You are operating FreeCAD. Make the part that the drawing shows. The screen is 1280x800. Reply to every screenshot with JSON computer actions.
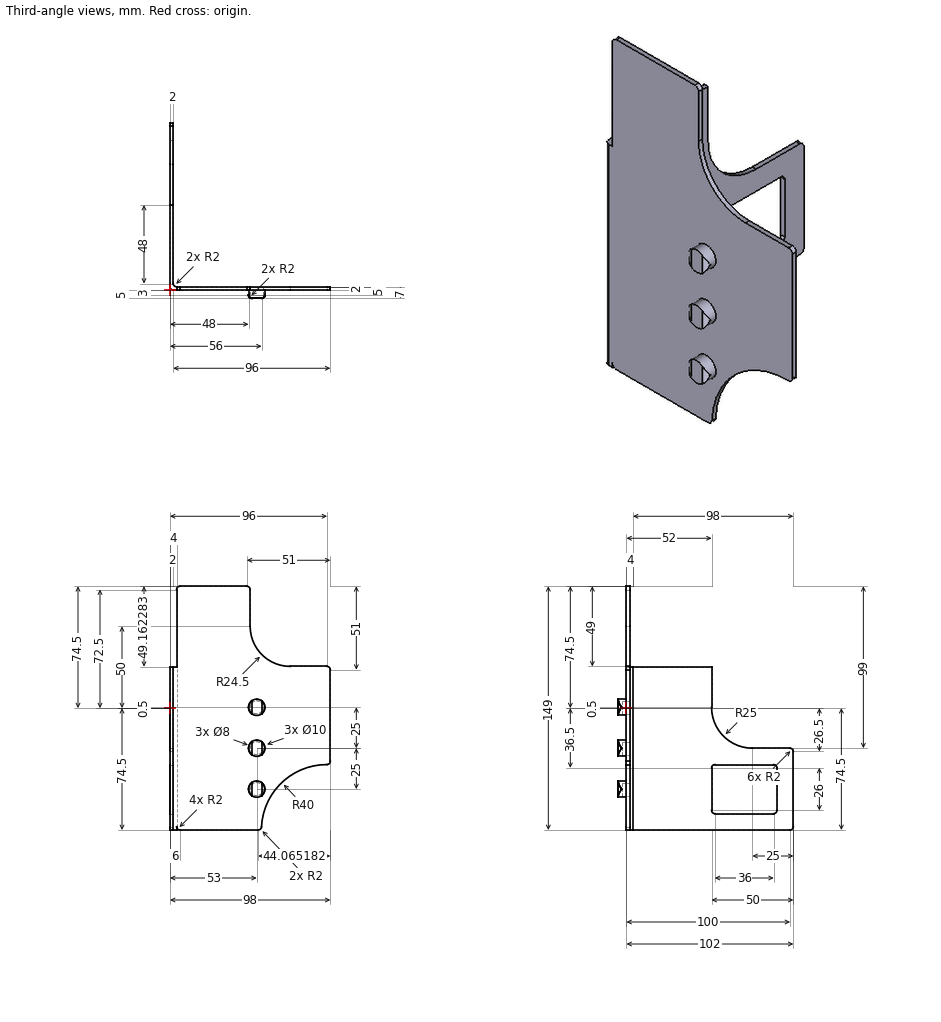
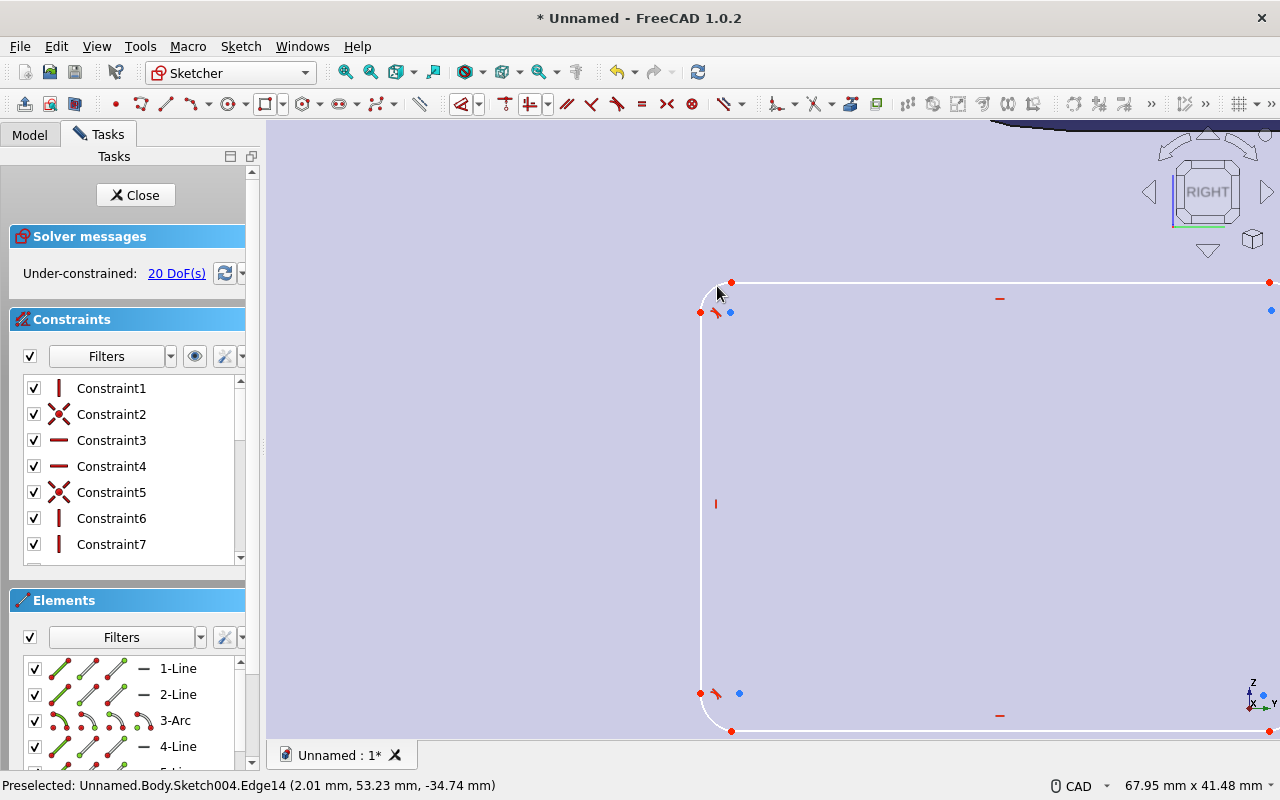
{"action": "scroll", "coordinate": [714, 492], "scroll_direction": "down", "scroll_amount": 5}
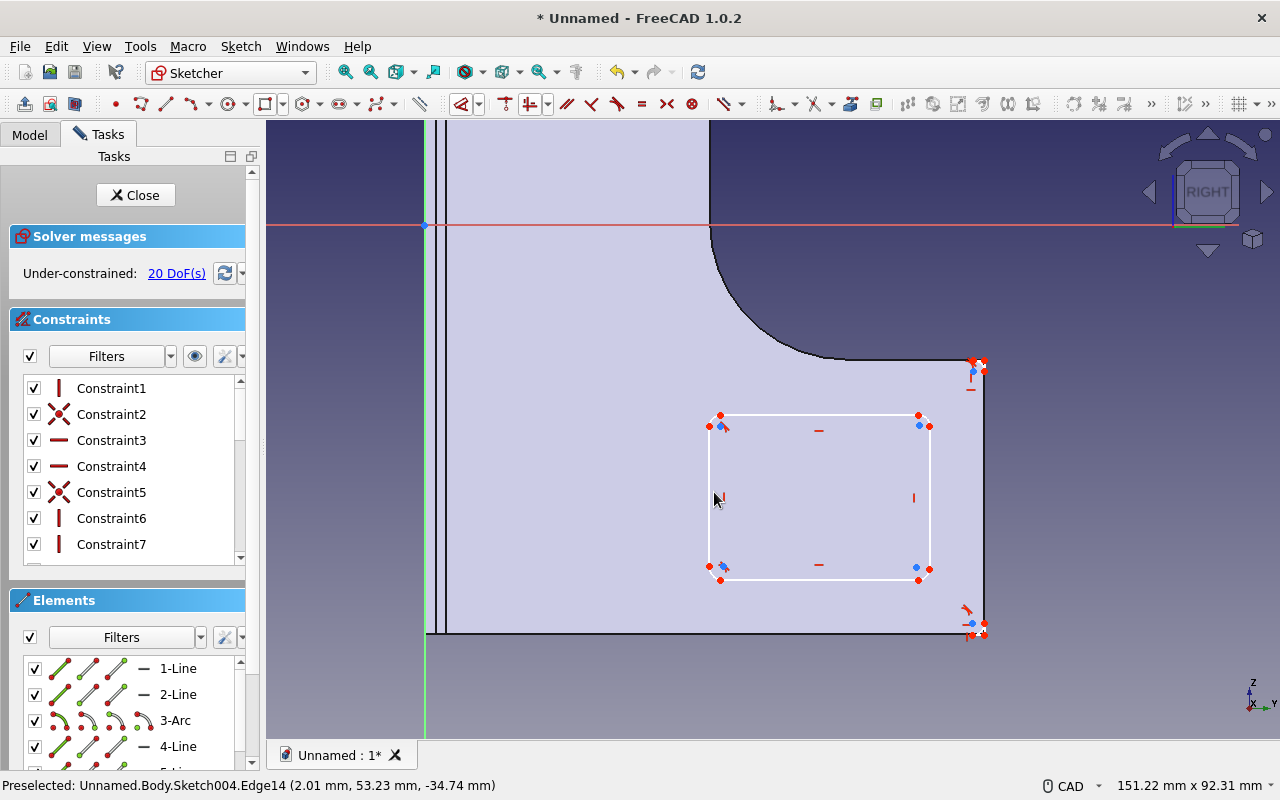
{"action": "left_click", "coordinate": [780, 580]}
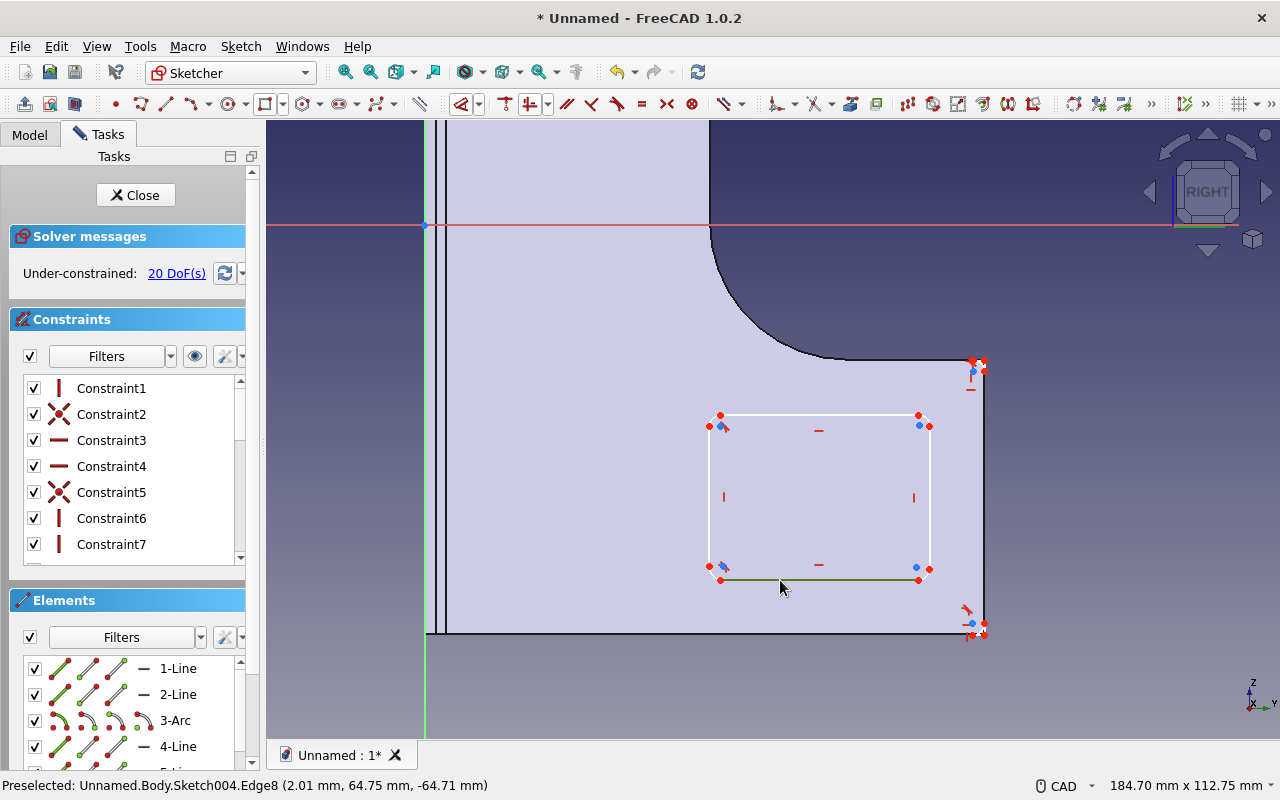
{"action": "scroll", "coordinate": [713, 575], "scroll_direction": "up", "scroll_amount": 2}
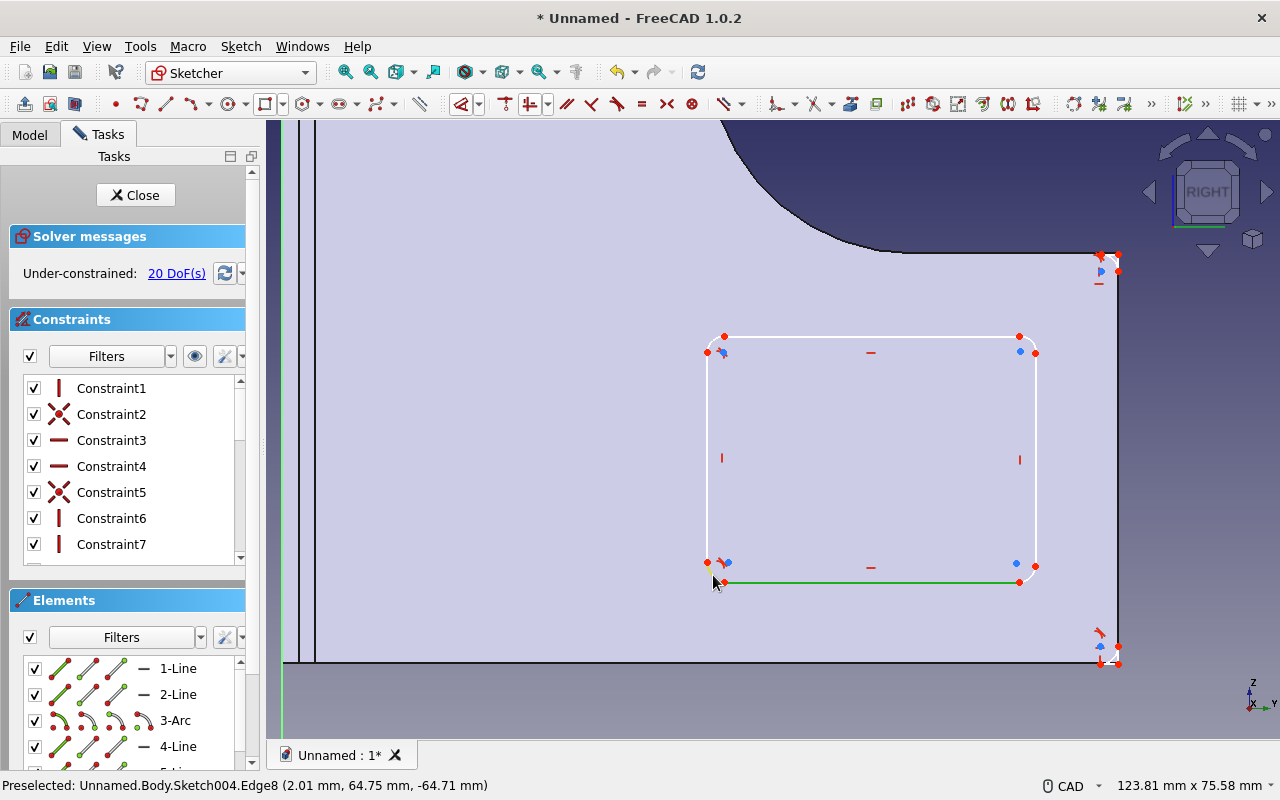
{"action": "left_click", "coordinate": [712, 575]}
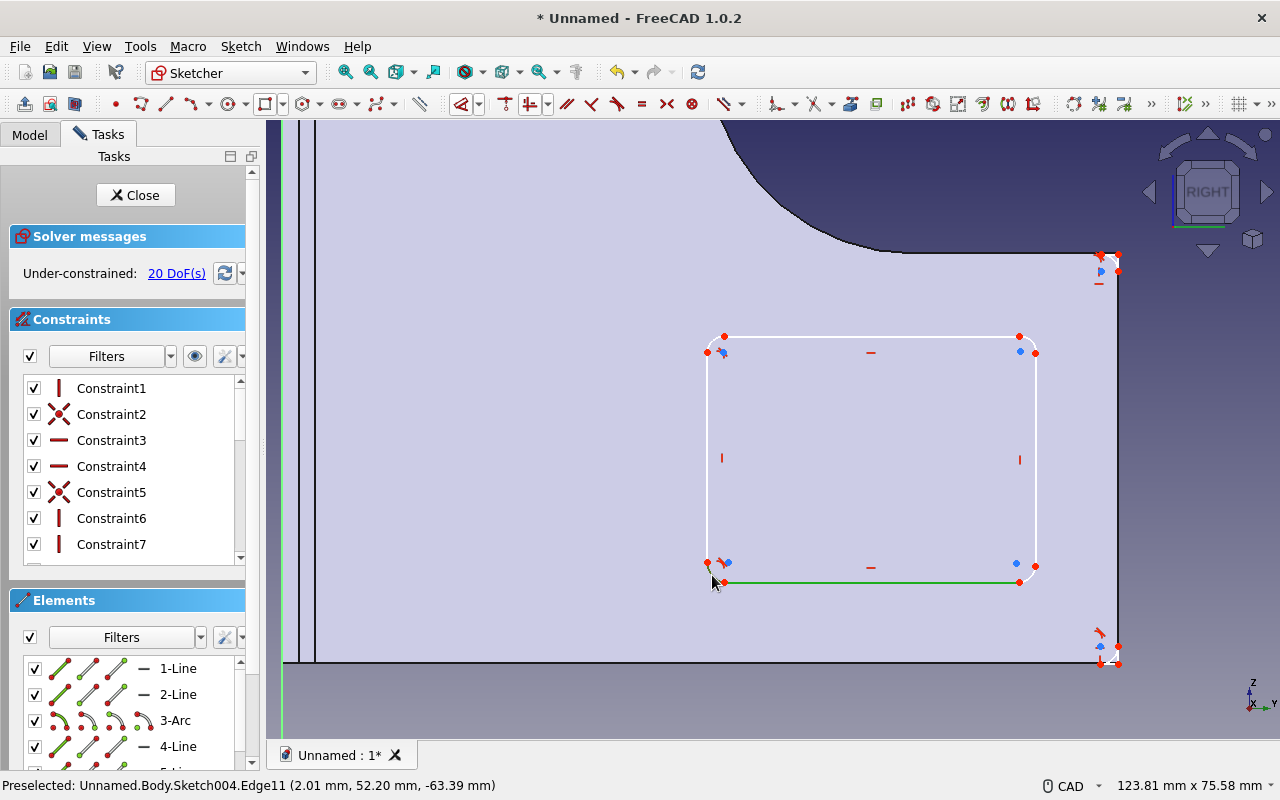
{"action": "key", "text": "t"}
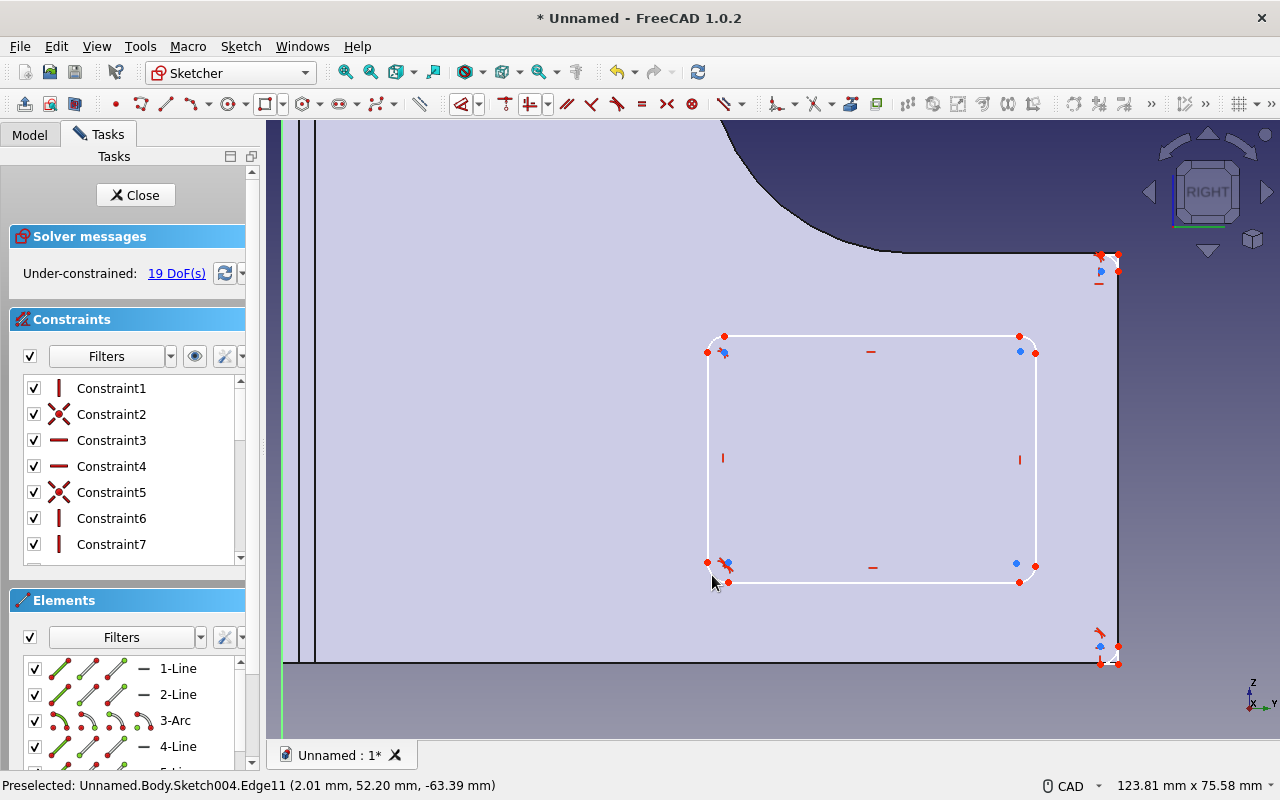
{"action": "left_click", "coordinate": [816, 583]}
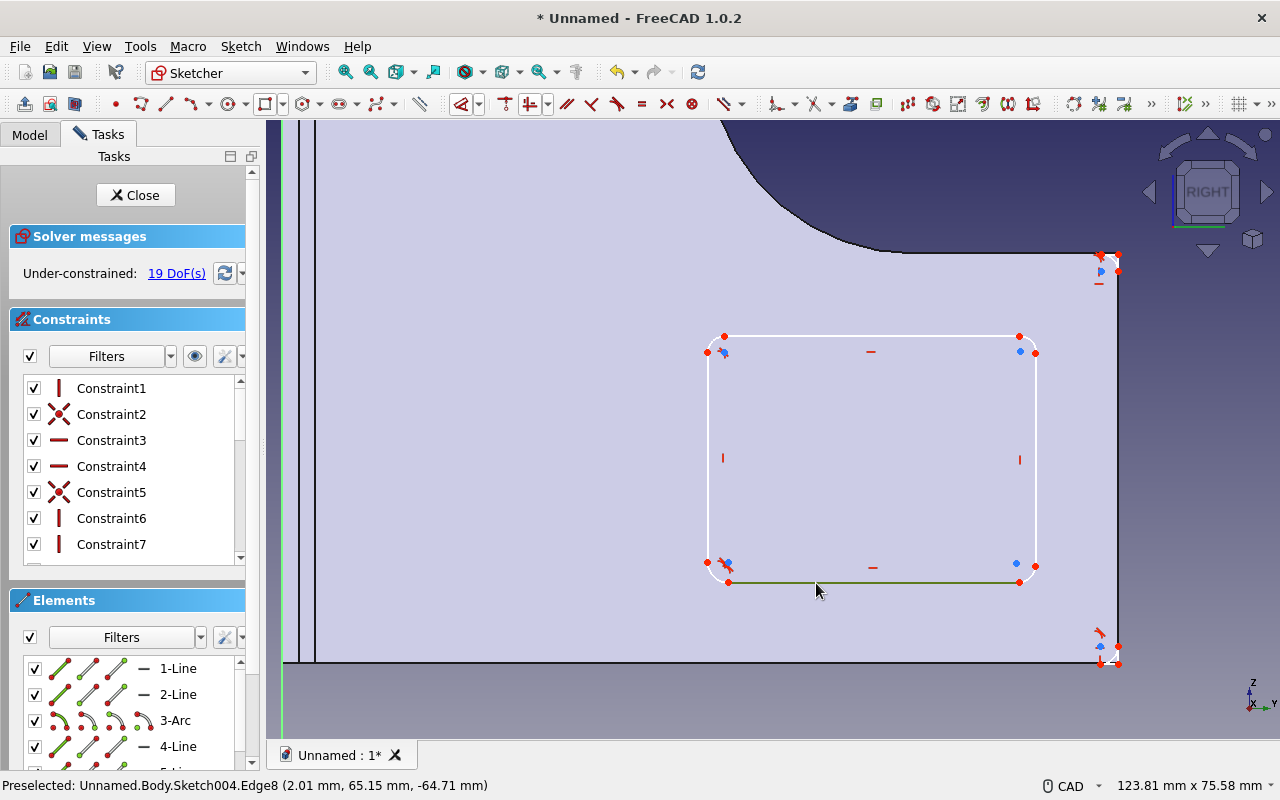
{"action": "left_click", "coordinate": [1030, 577]}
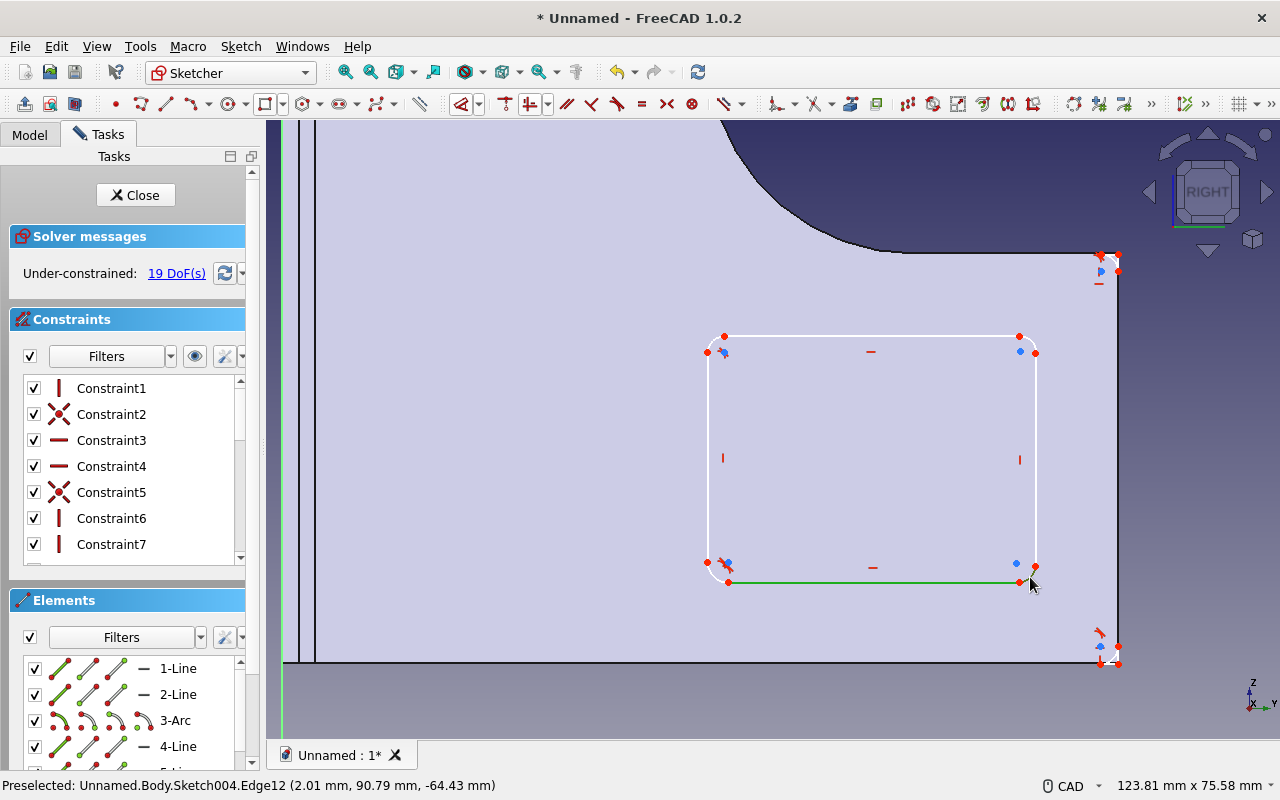
{"action": "key", "text": "t"}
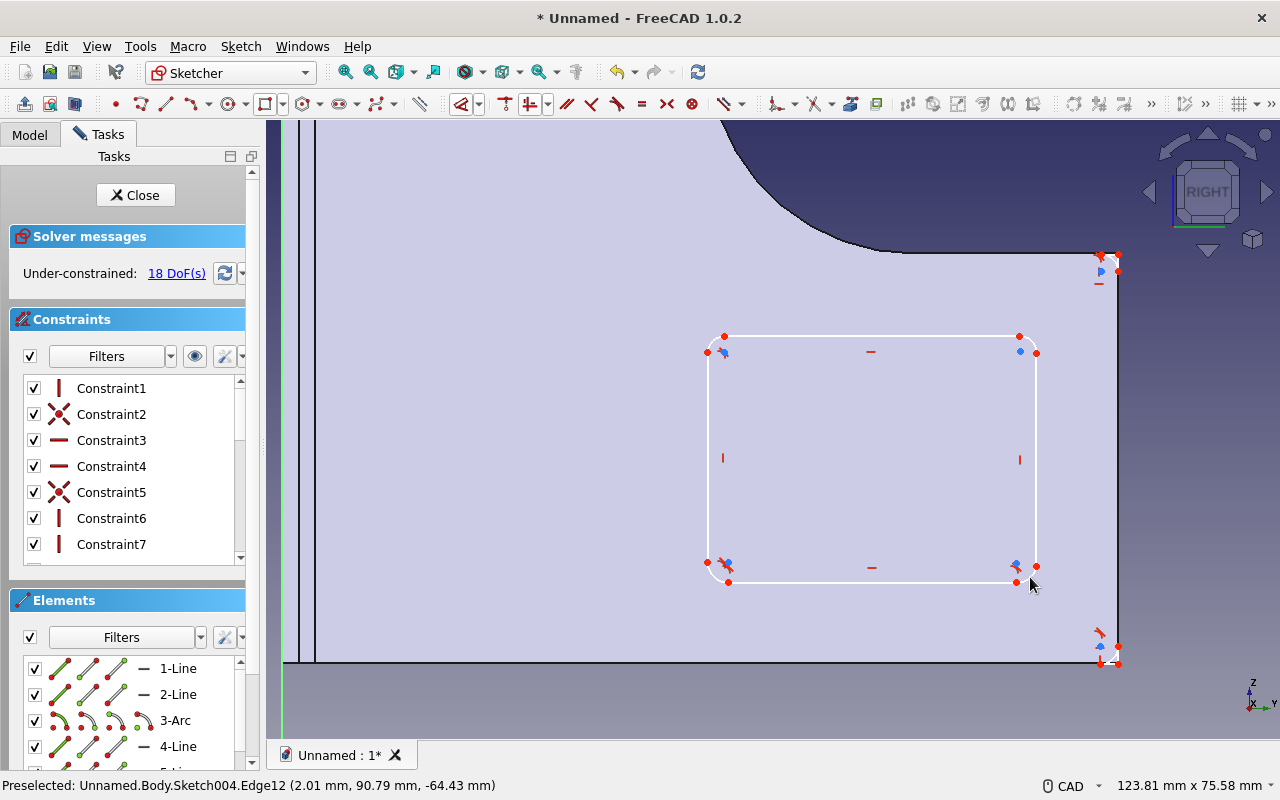
{"action": "left_click", "coordinate": [1036, 502]}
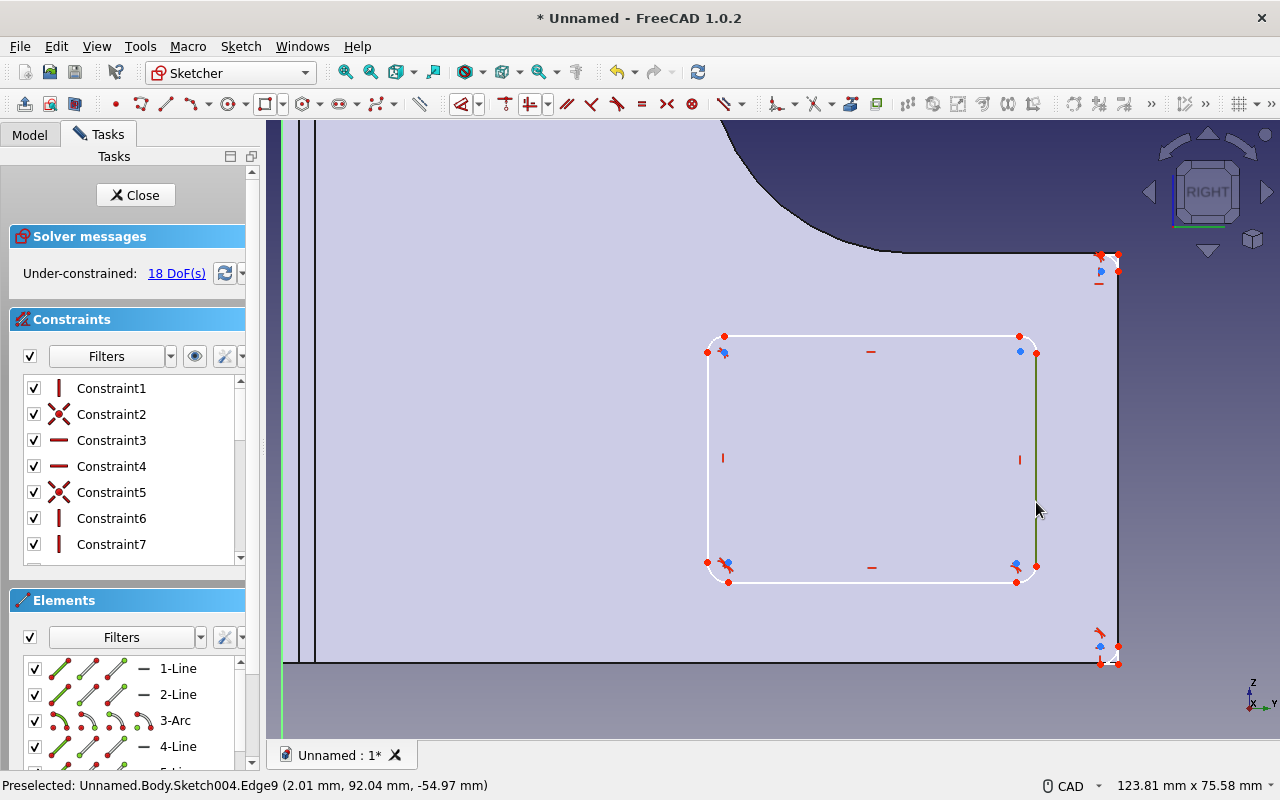
{"action": "left_click", "coordinate": [1030, 578]}